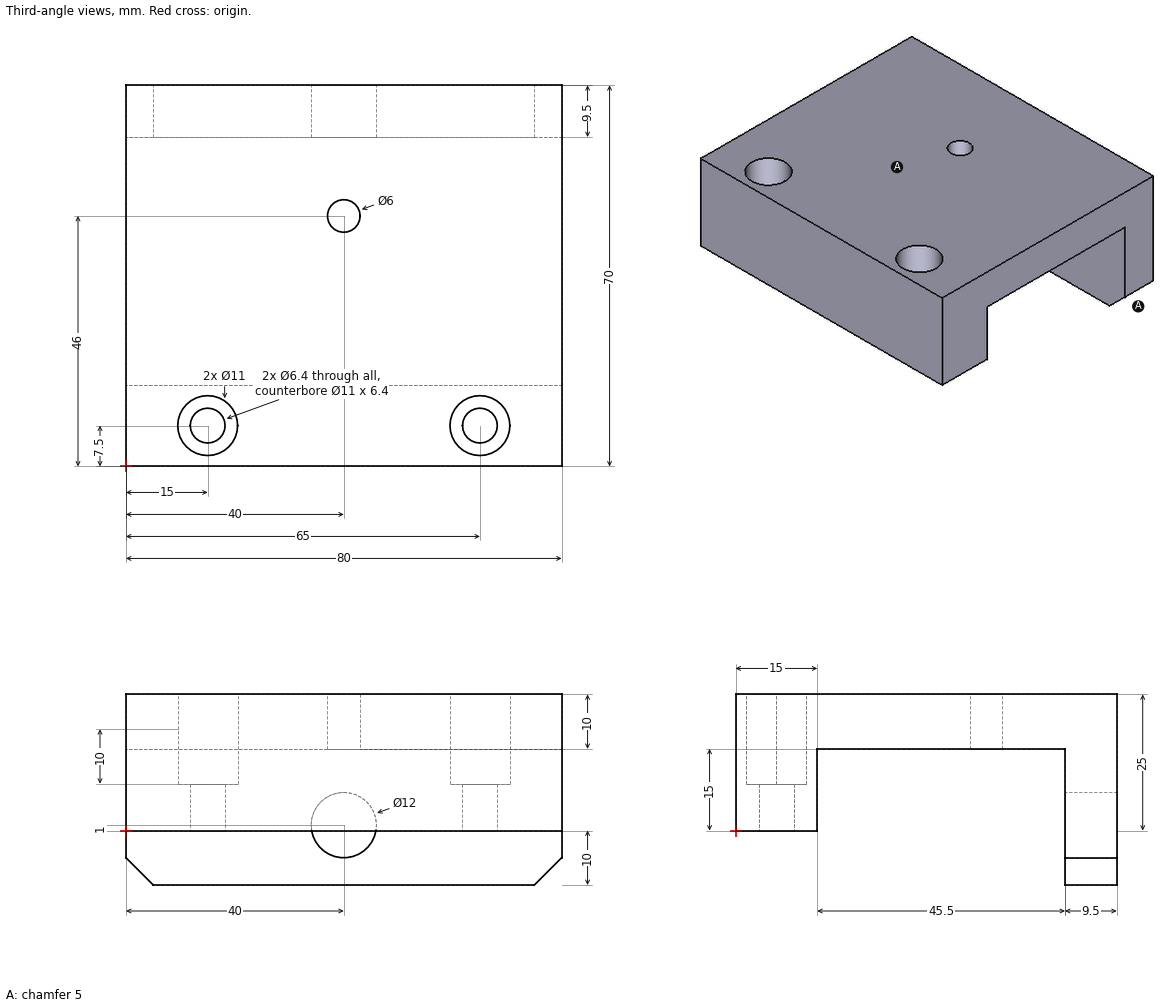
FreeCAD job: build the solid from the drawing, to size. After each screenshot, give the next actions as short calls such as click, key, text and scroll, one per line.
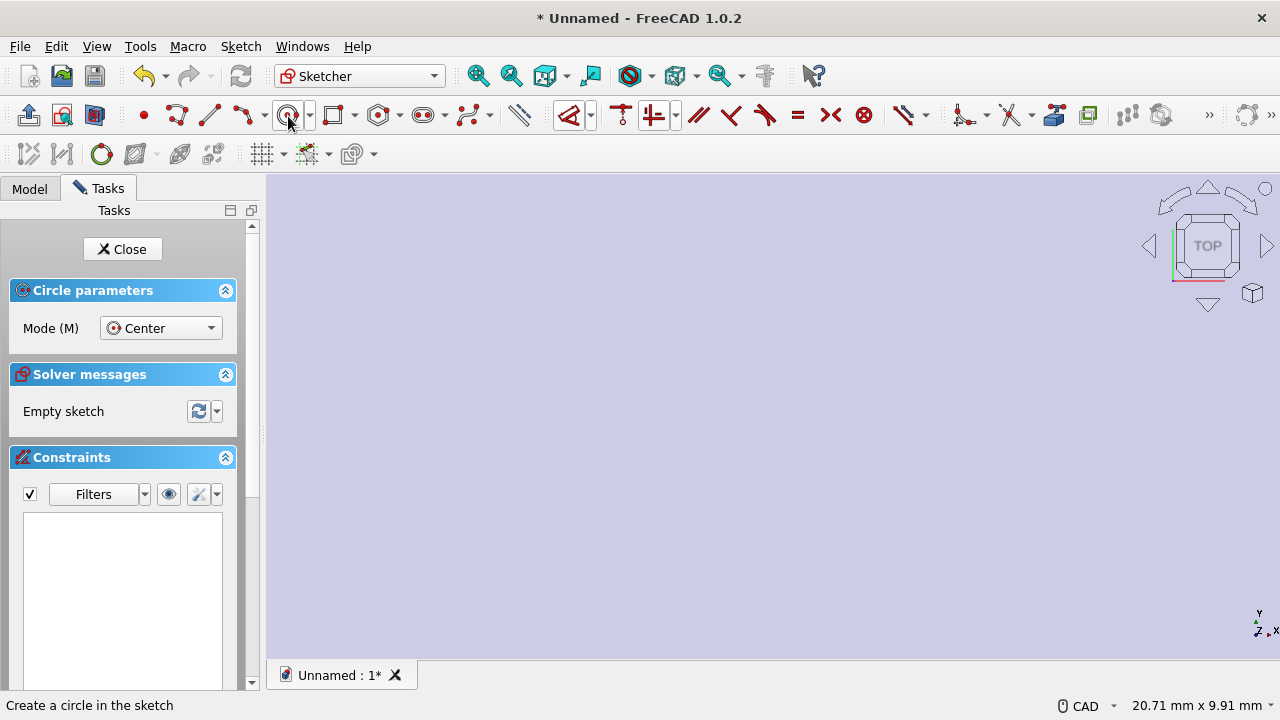
click(698, 410)
move(802, 306)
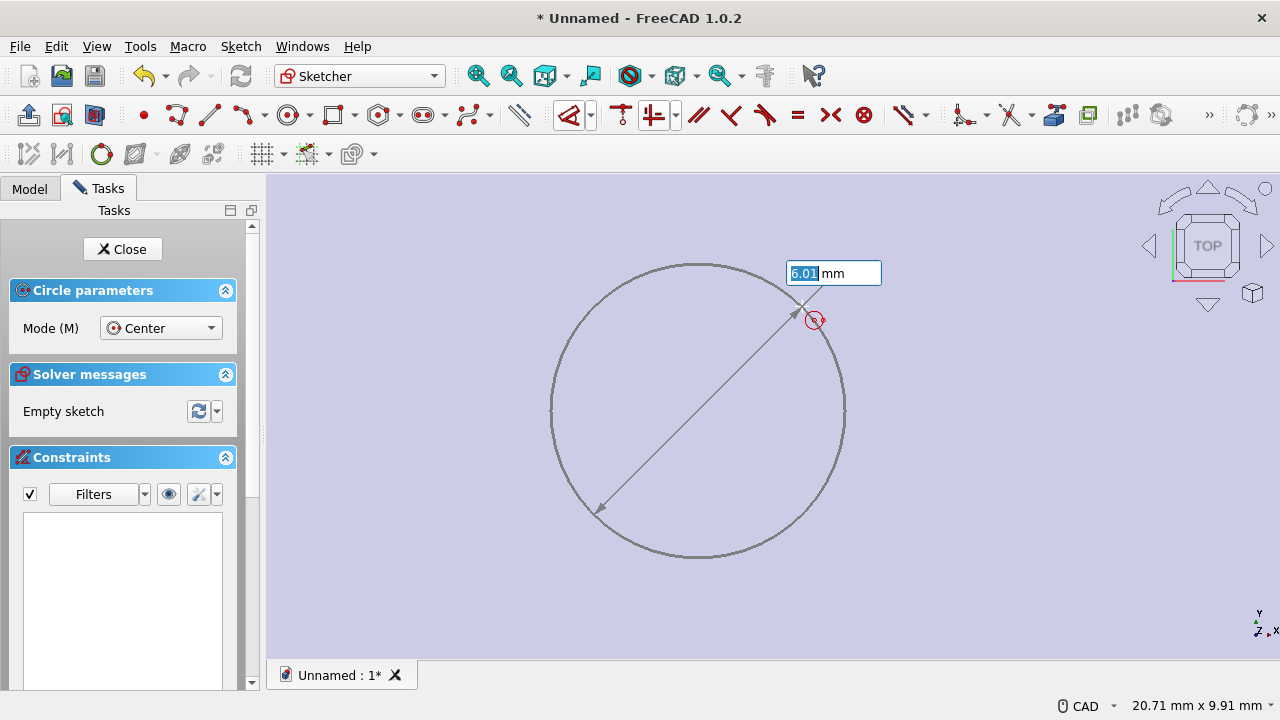
text(6)
key(Return)
key(Escape)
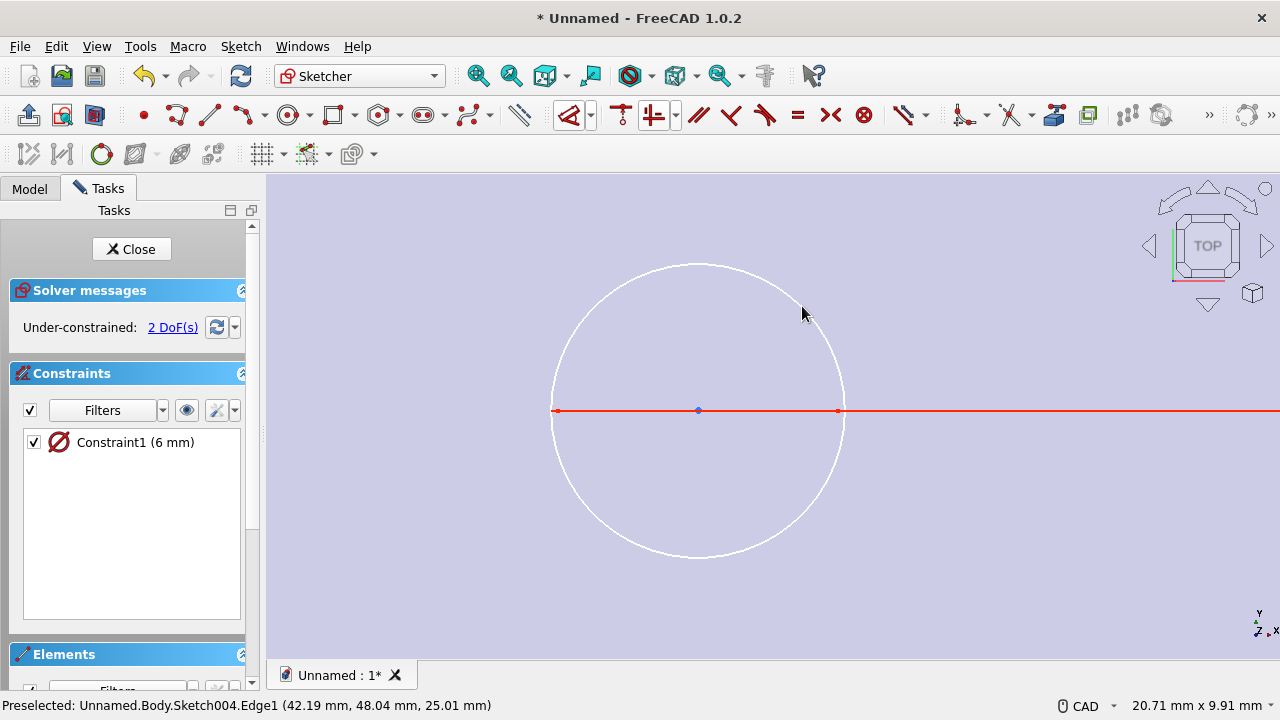
click(698, 411)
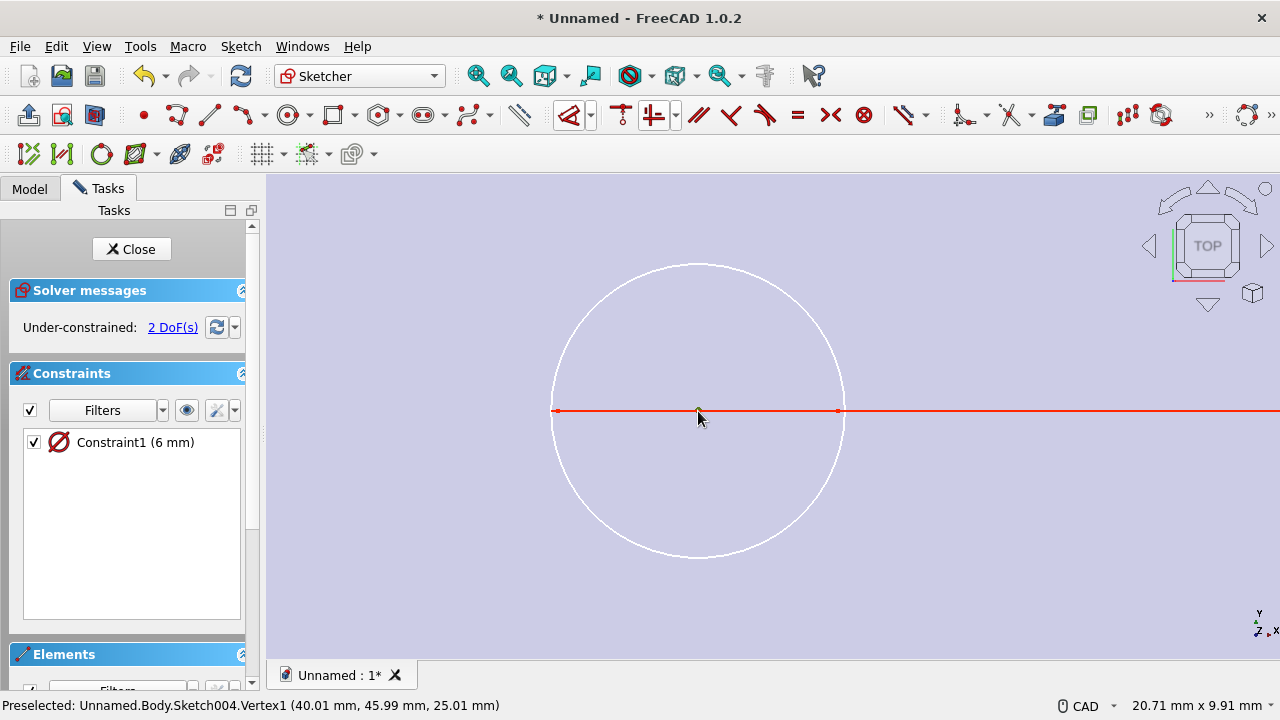
key(l)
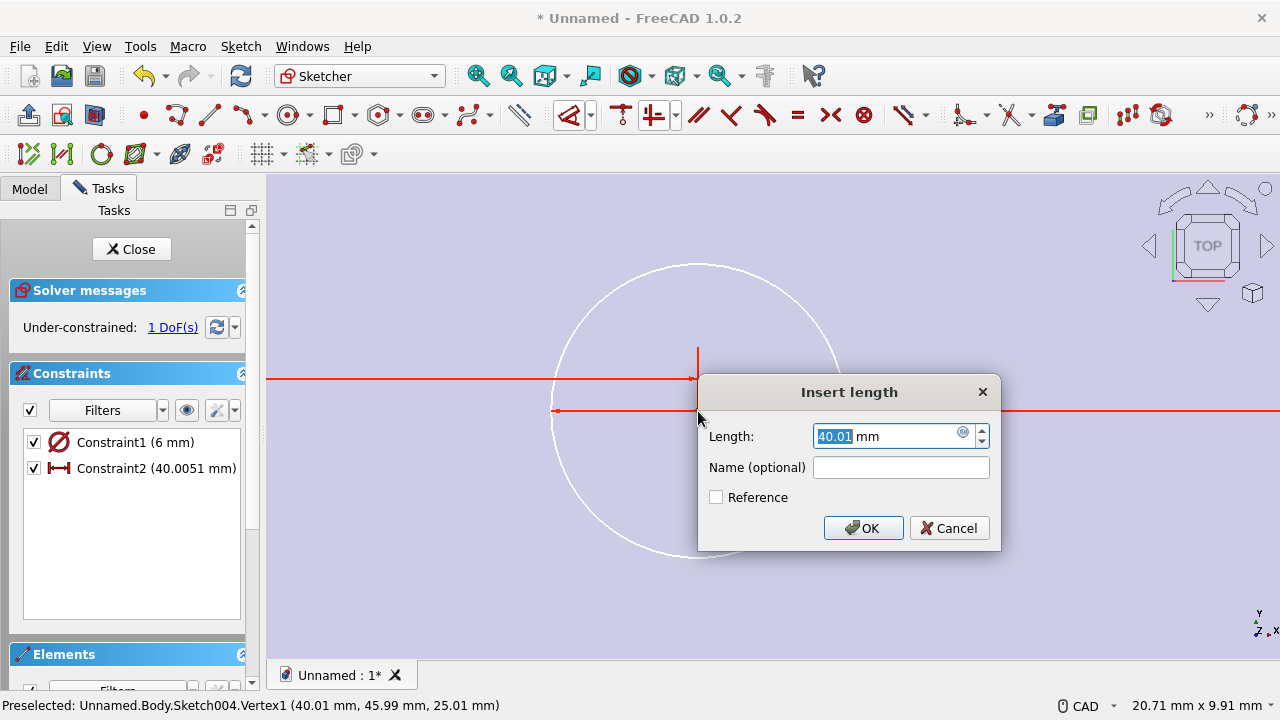
text(40)
key(Return)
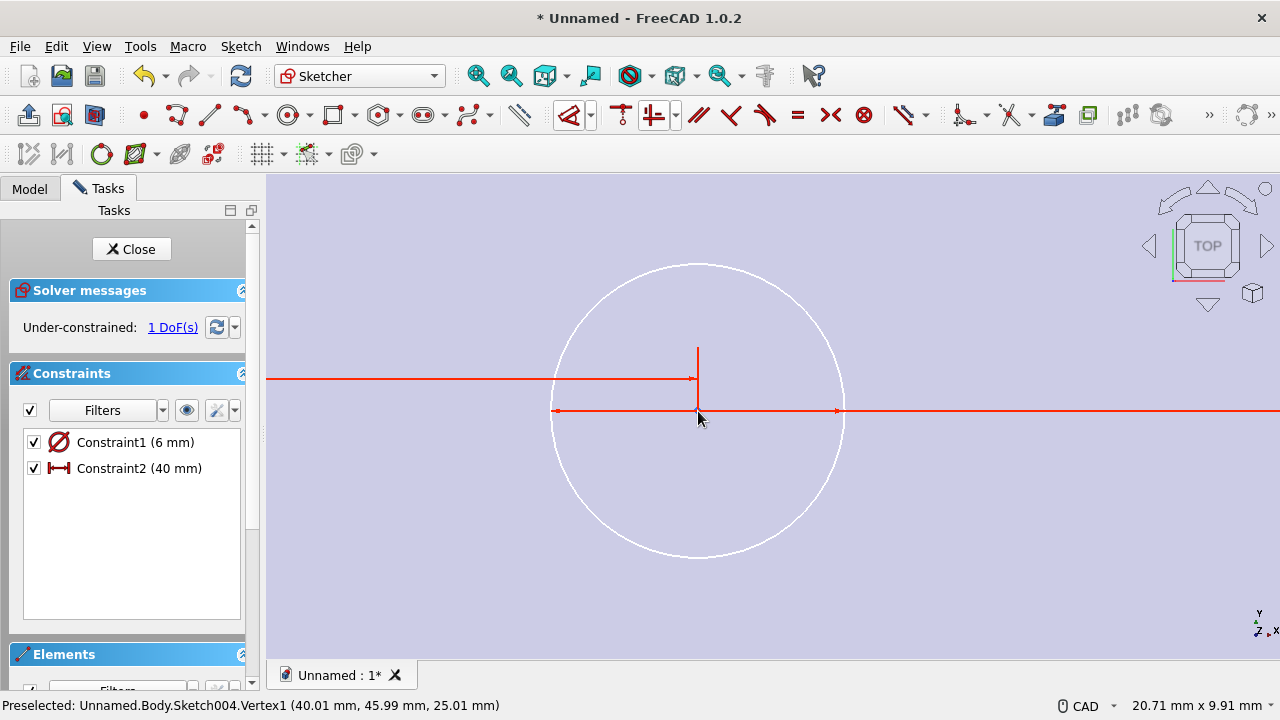
click(698, 411)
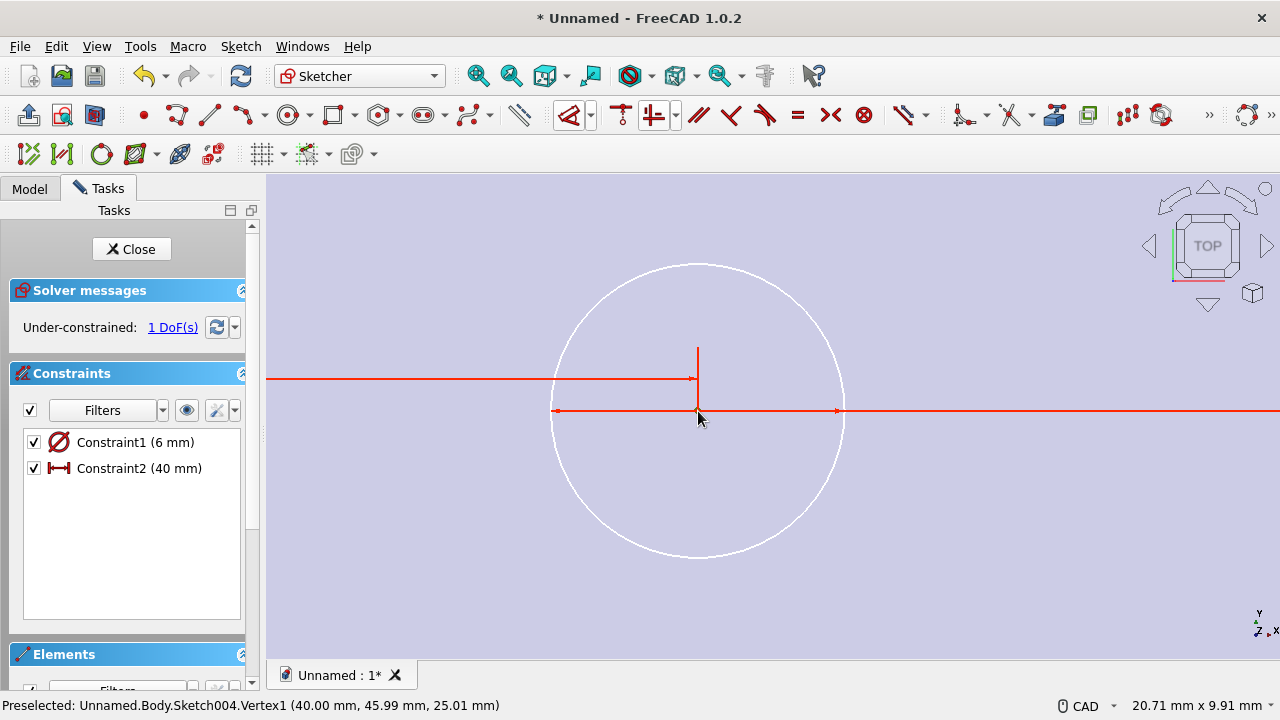
click(590, 116)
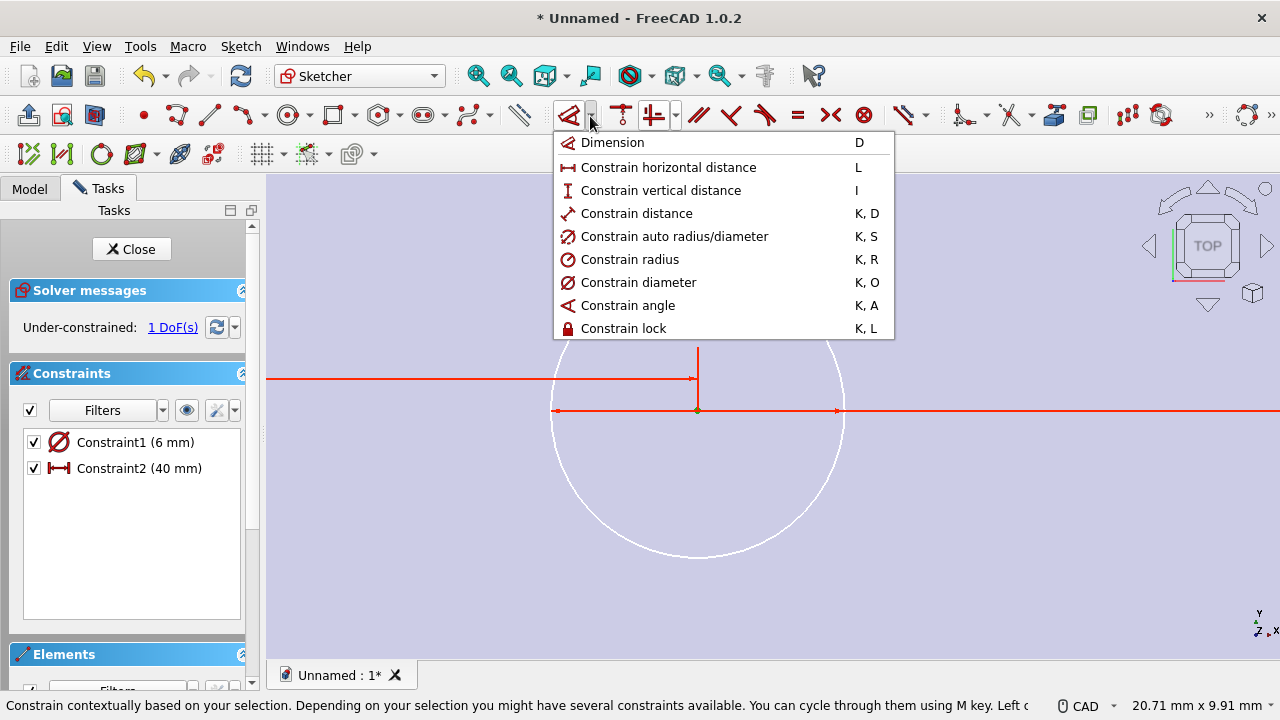
click(724, 190)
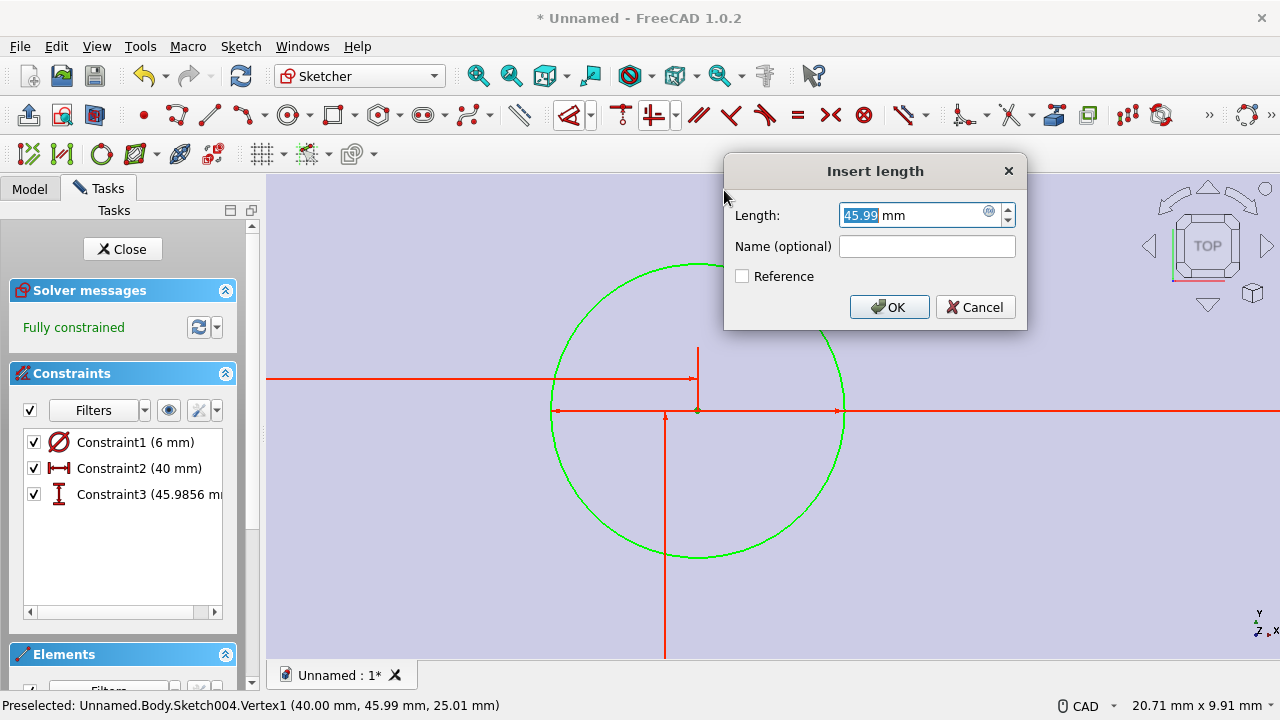
text(46)
key(Return)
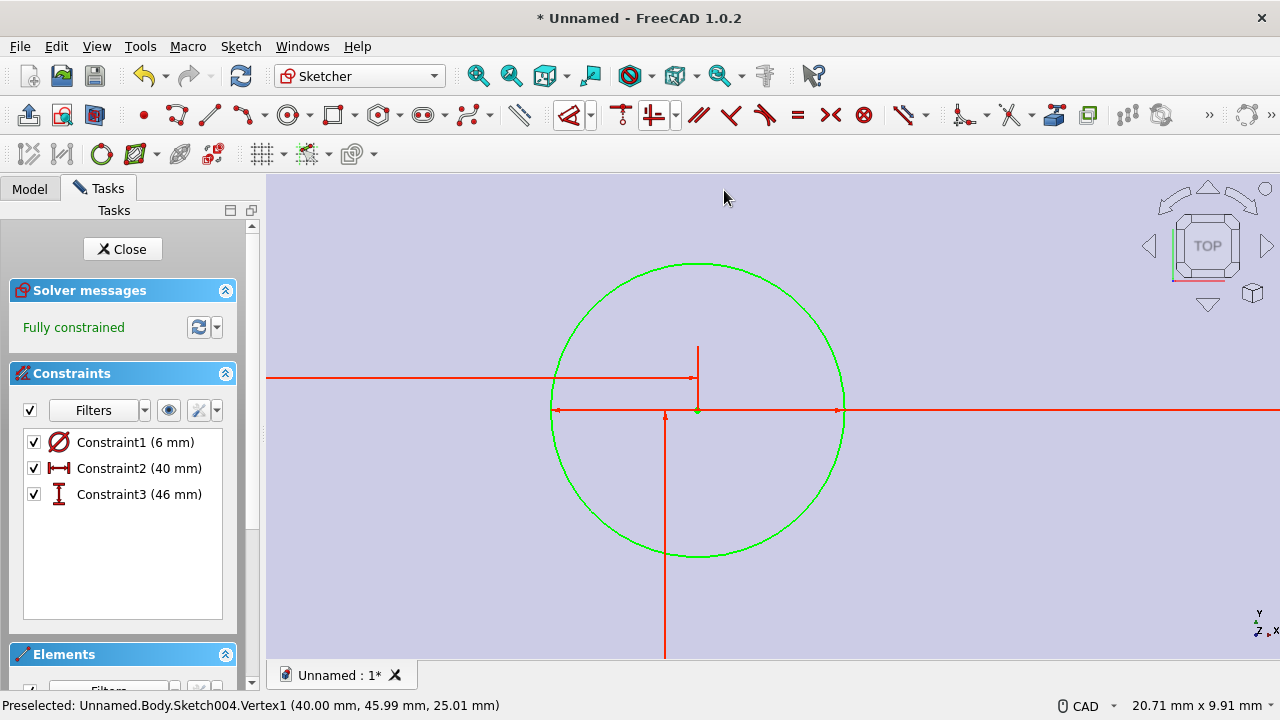
click(123, 249)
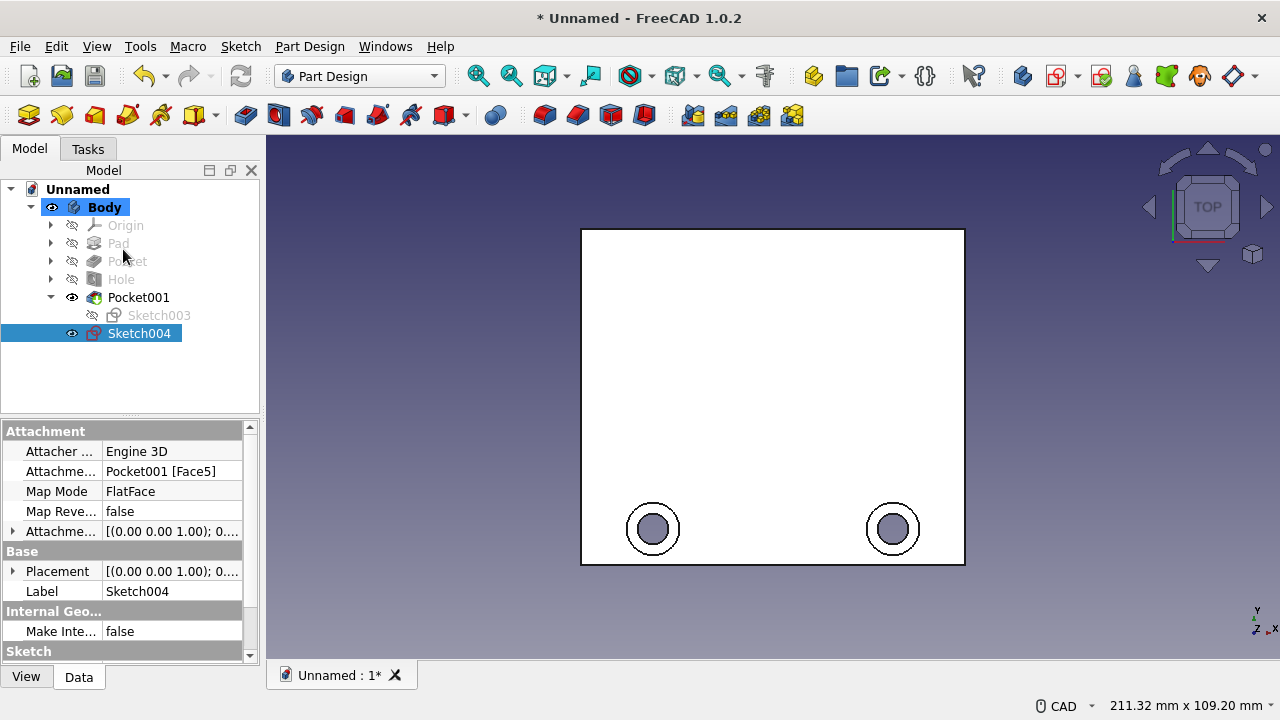
click(246, 116)